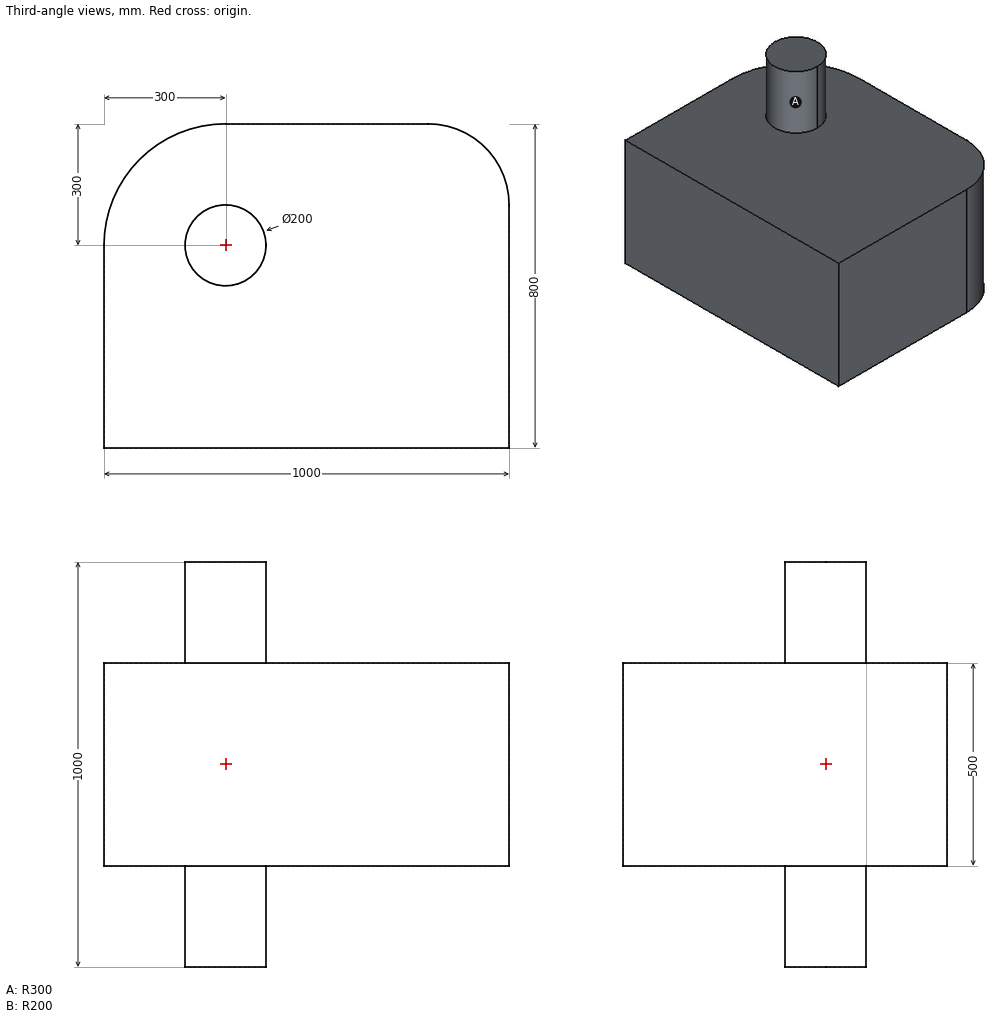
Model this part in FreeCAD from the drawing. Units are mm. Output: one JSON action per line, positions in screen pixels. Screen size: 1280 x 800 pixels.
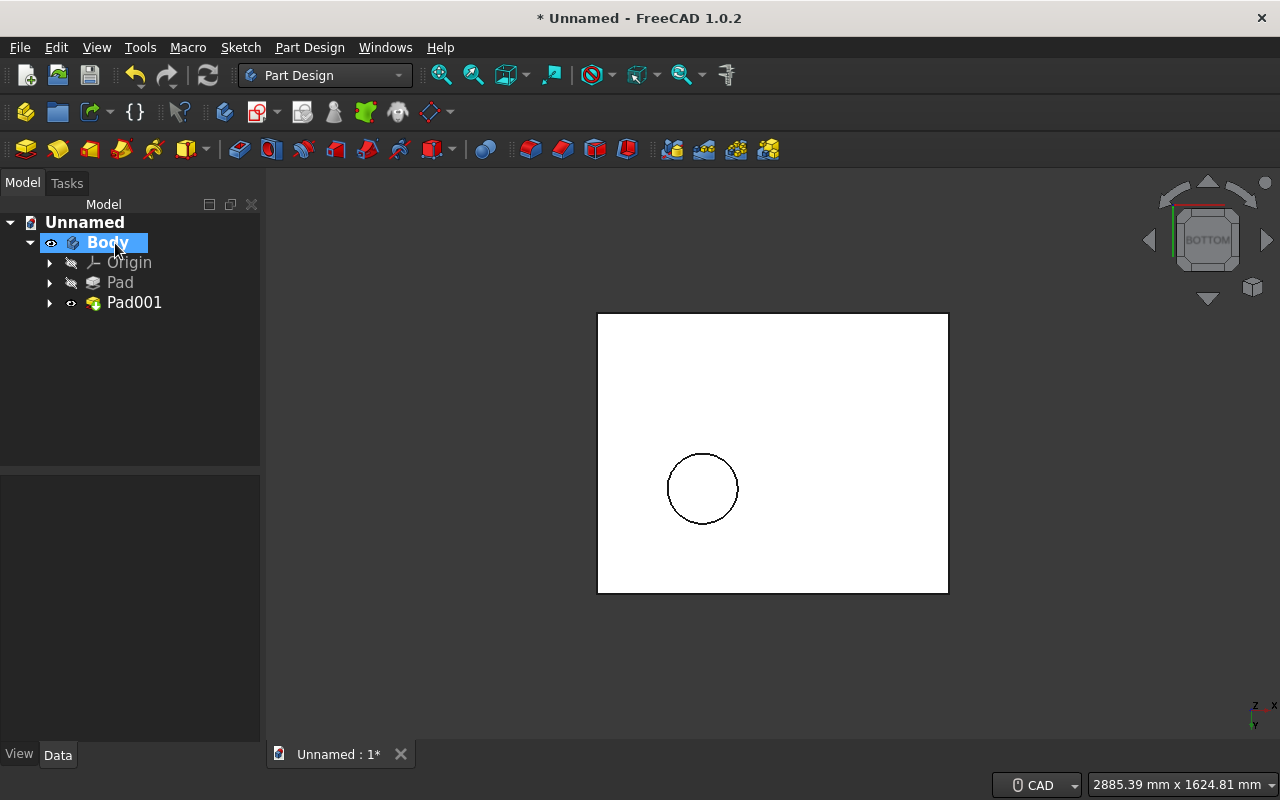
{"action": "key", "text": "4"}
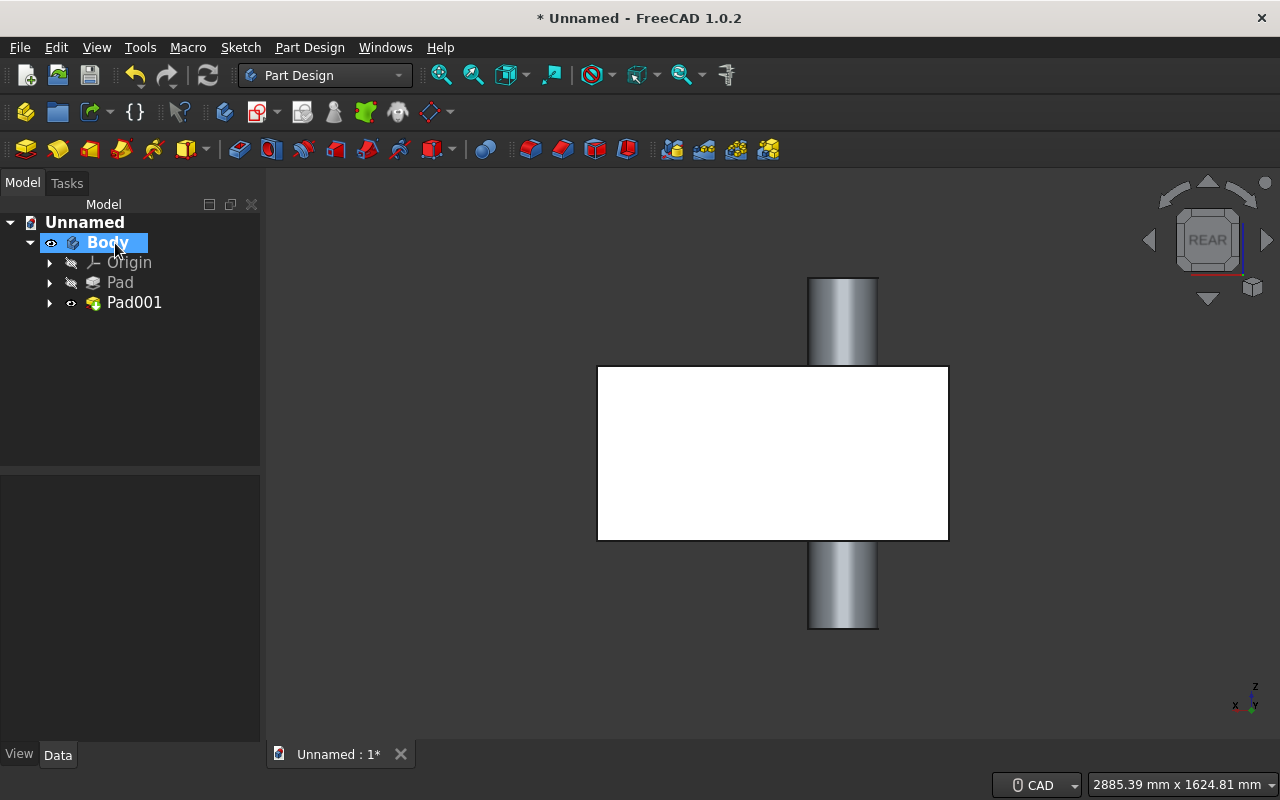
{"action": "left_click", "coordinate": [949, 452]}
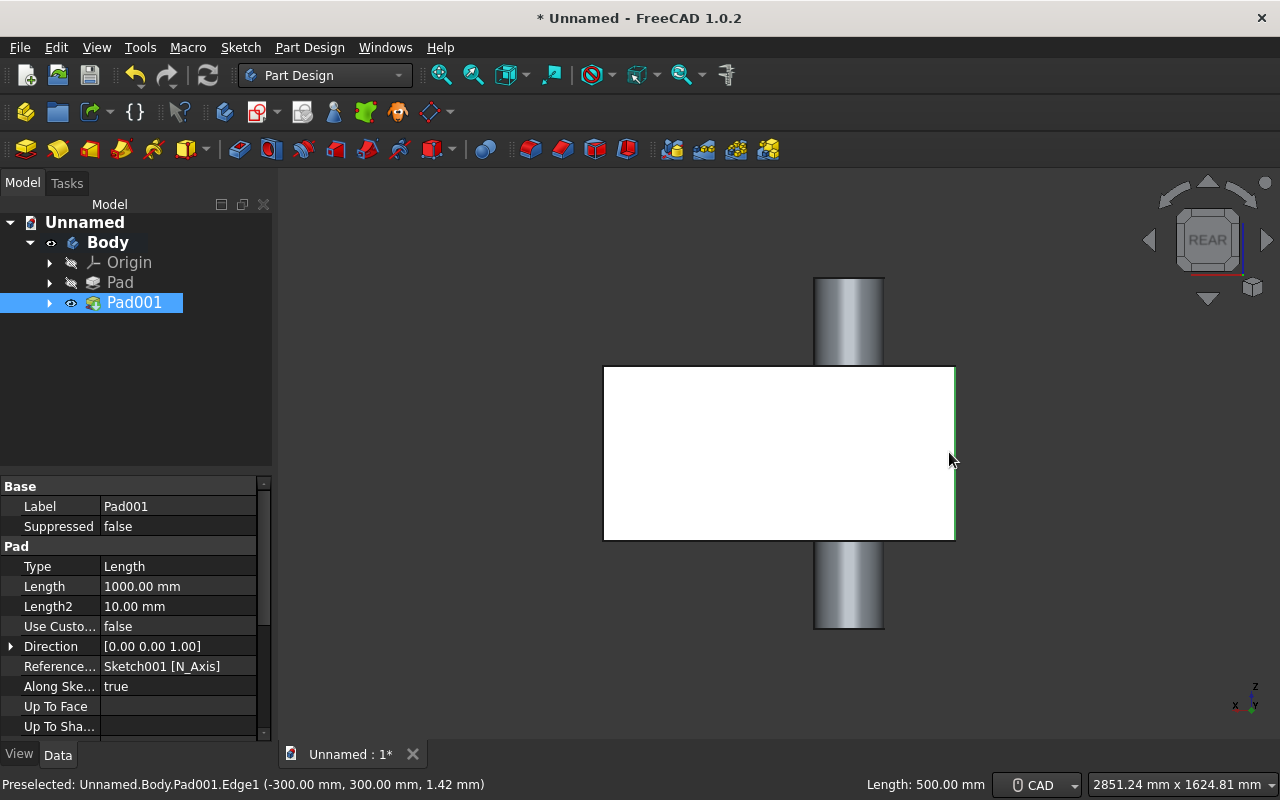
{"action": "left_click", "coordinate": [532, 150]}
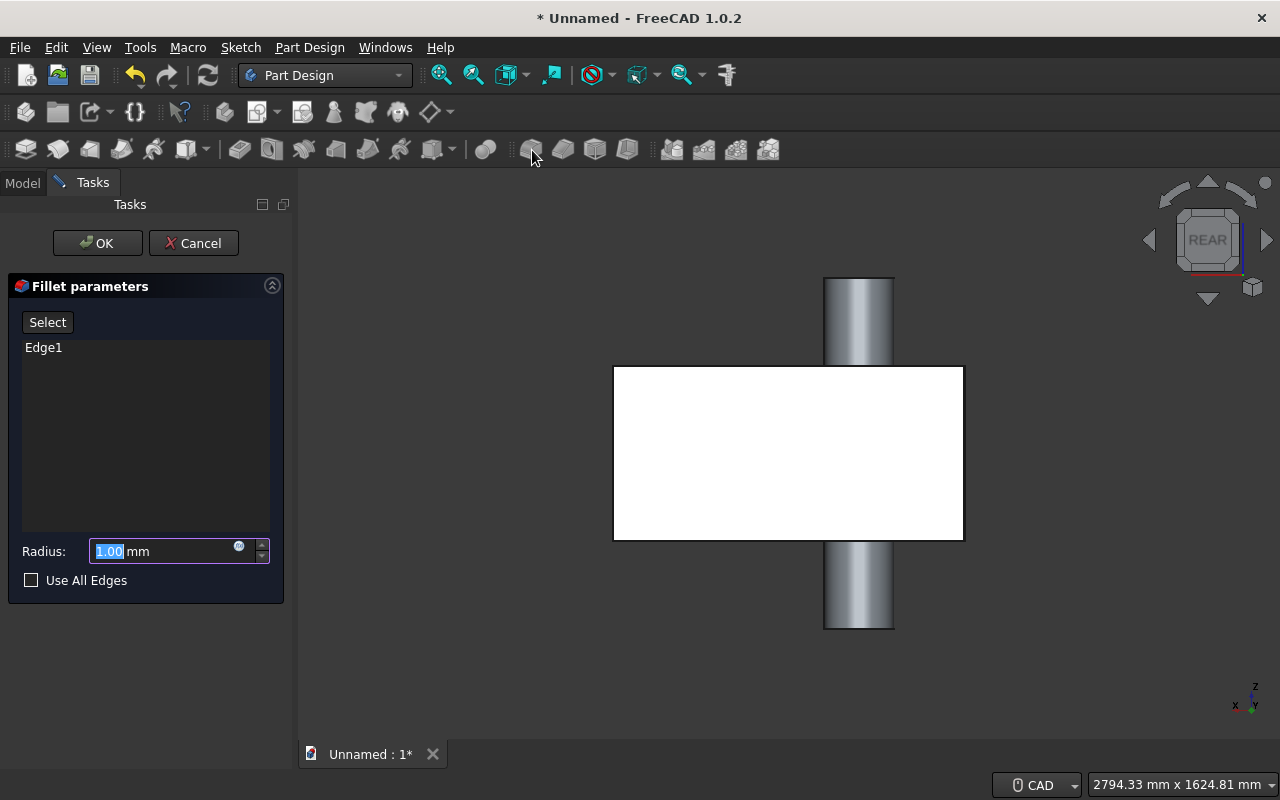
{"action": "type", "text": "300"}
{"action": "key", "text": "Tab"}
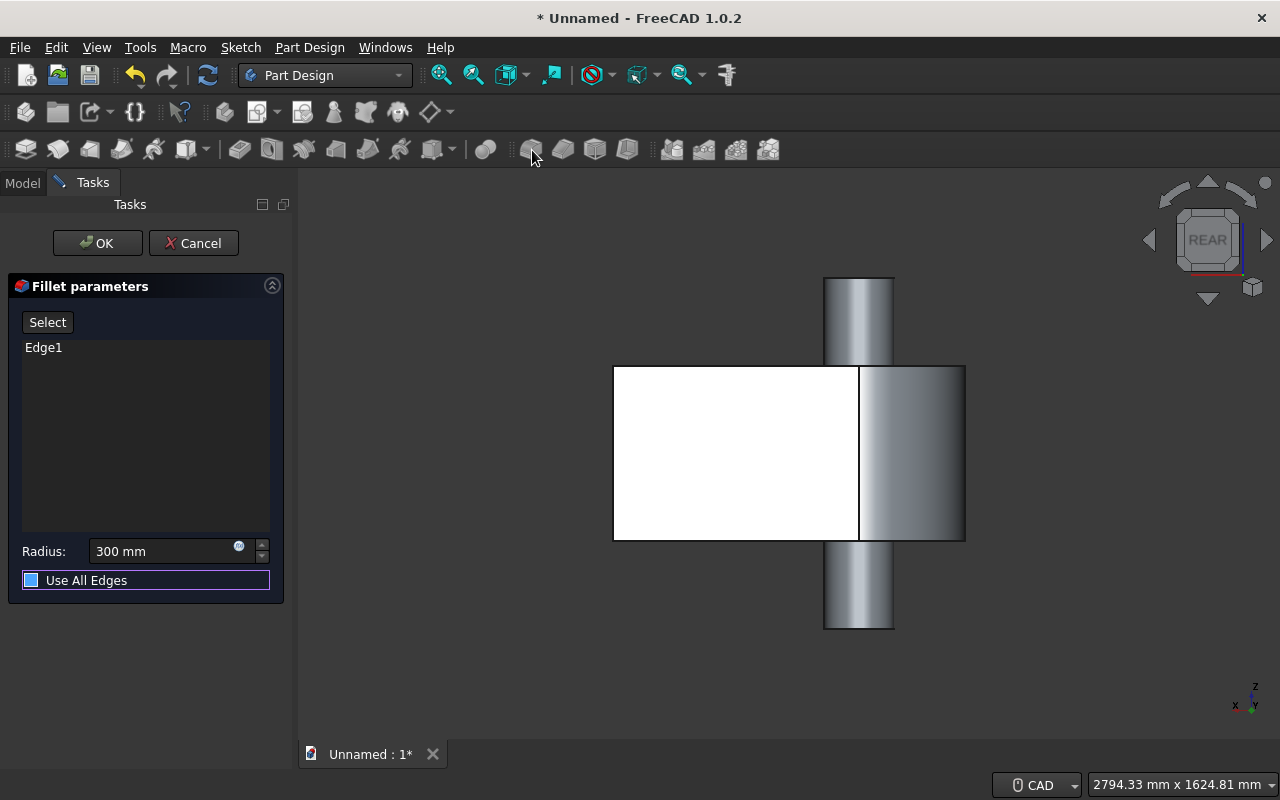
{"action": "left_click", "coordinate": [98, 243]}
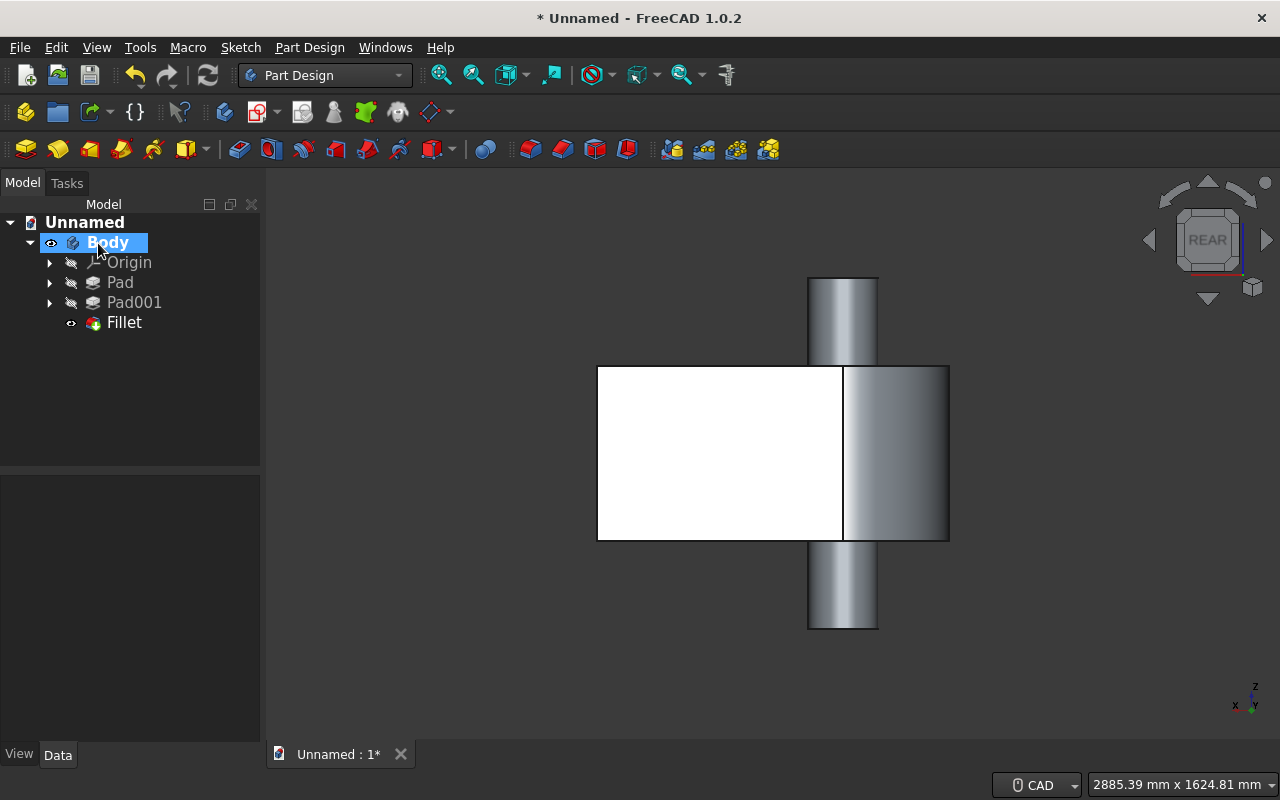
{"action": "left_click", "coordinate": [597, 452]}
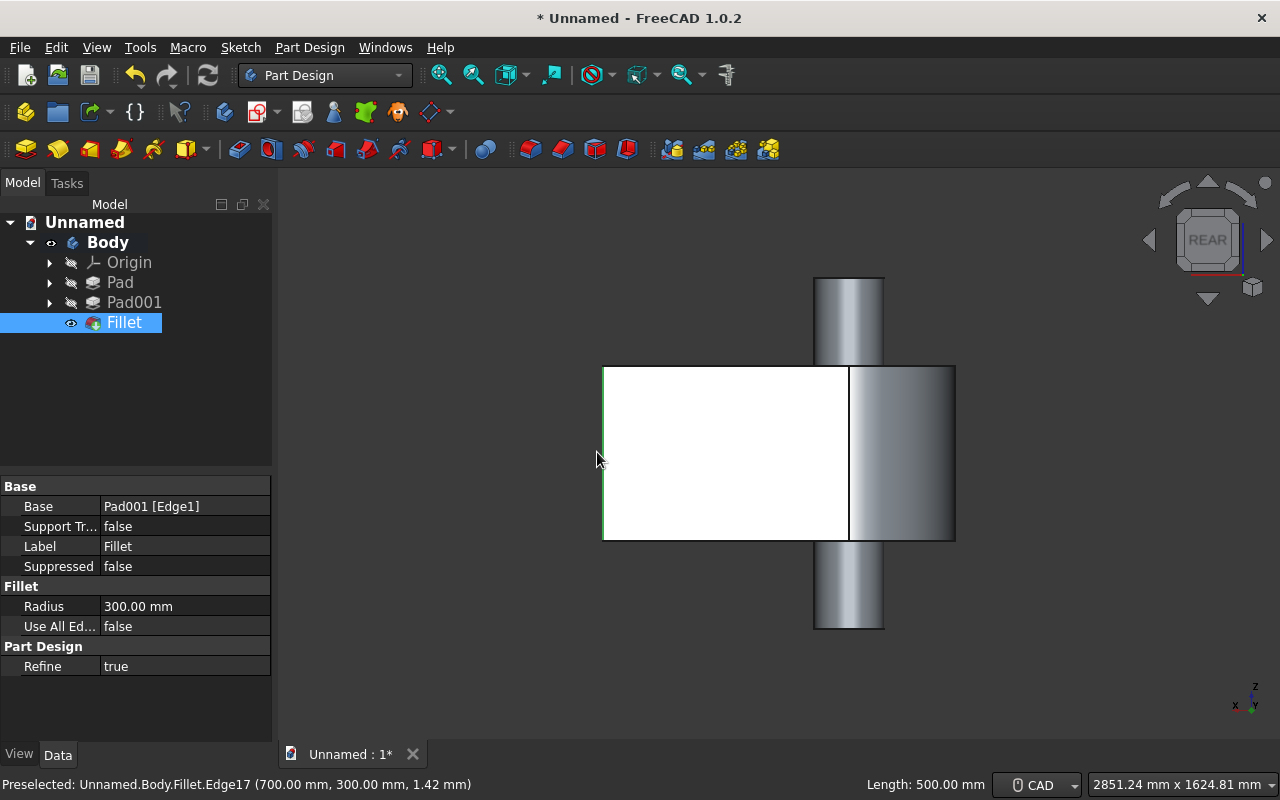
{"action": "left_click", "coordinate": [532, 150]}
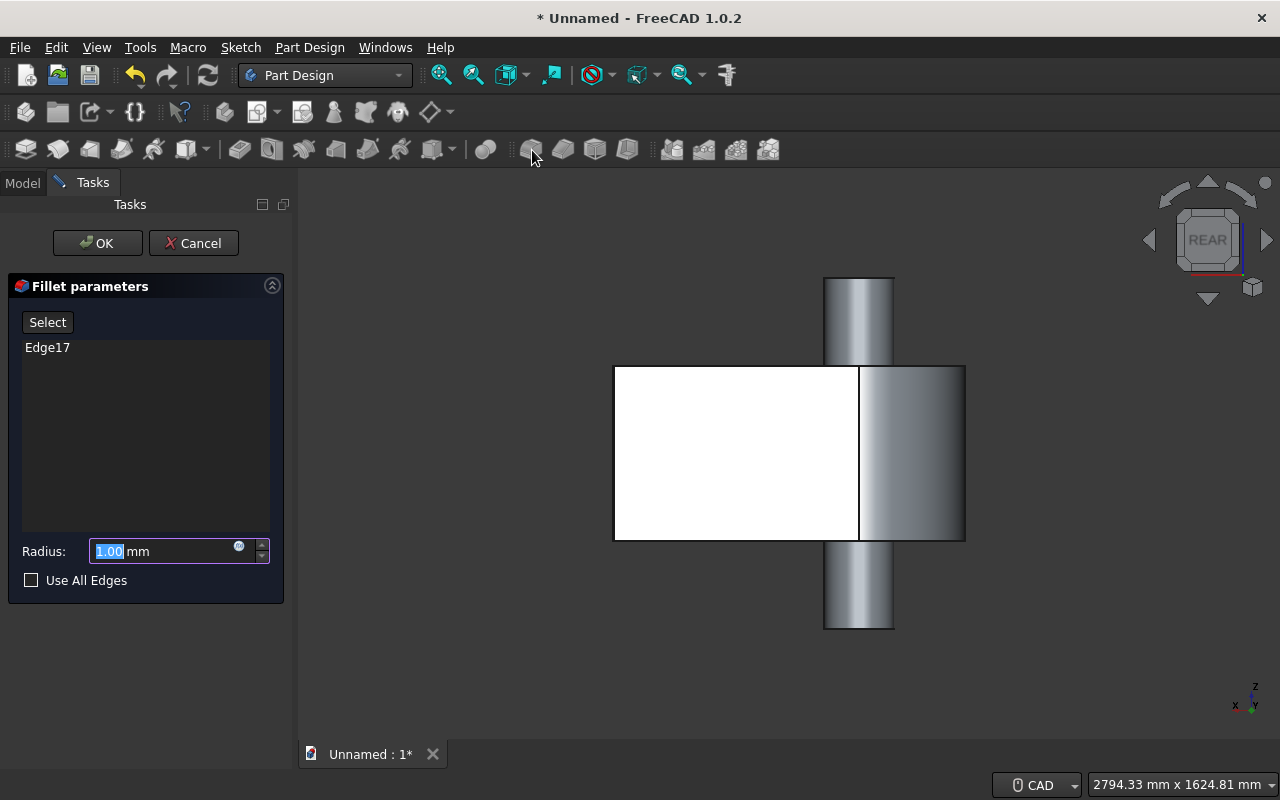
{"action": "type", "text": "200"}
{"action": "key", "text": "Tab"}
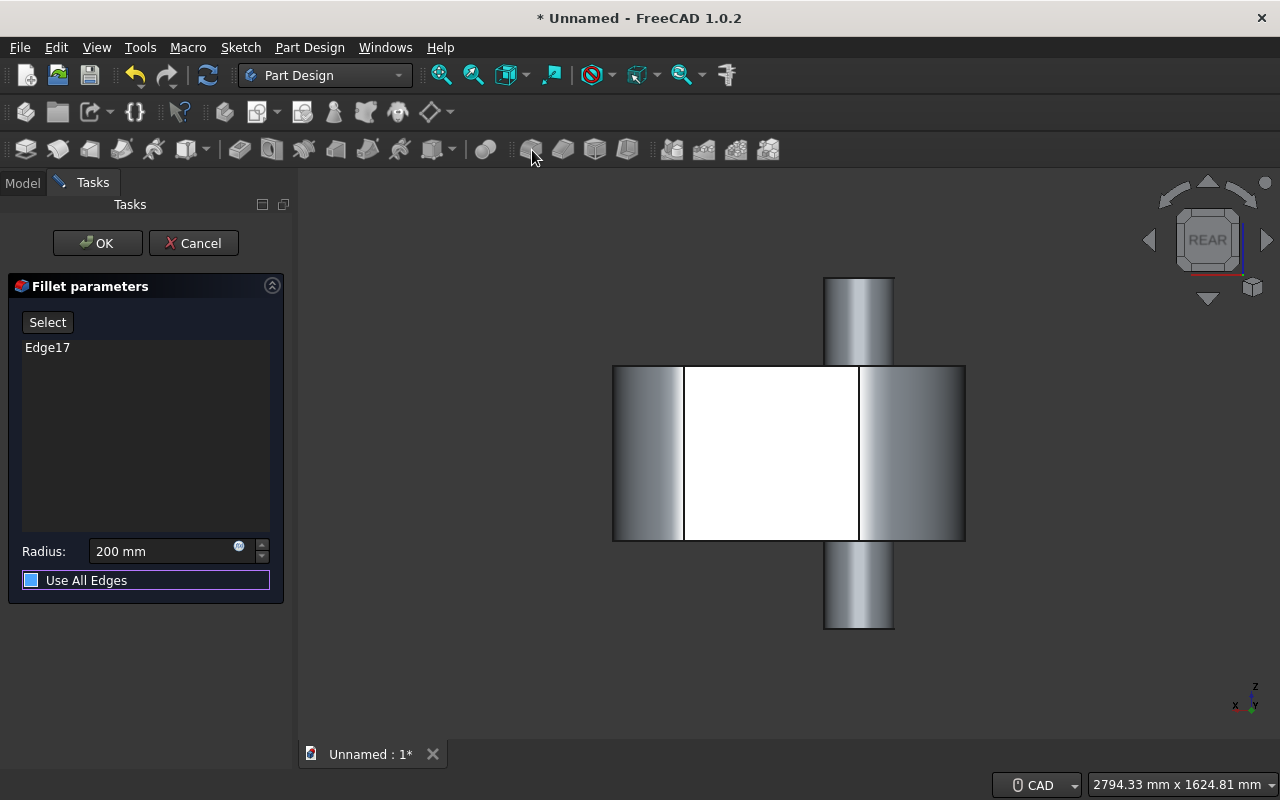
{"action": "left_click", "coordinate": [98, 243]}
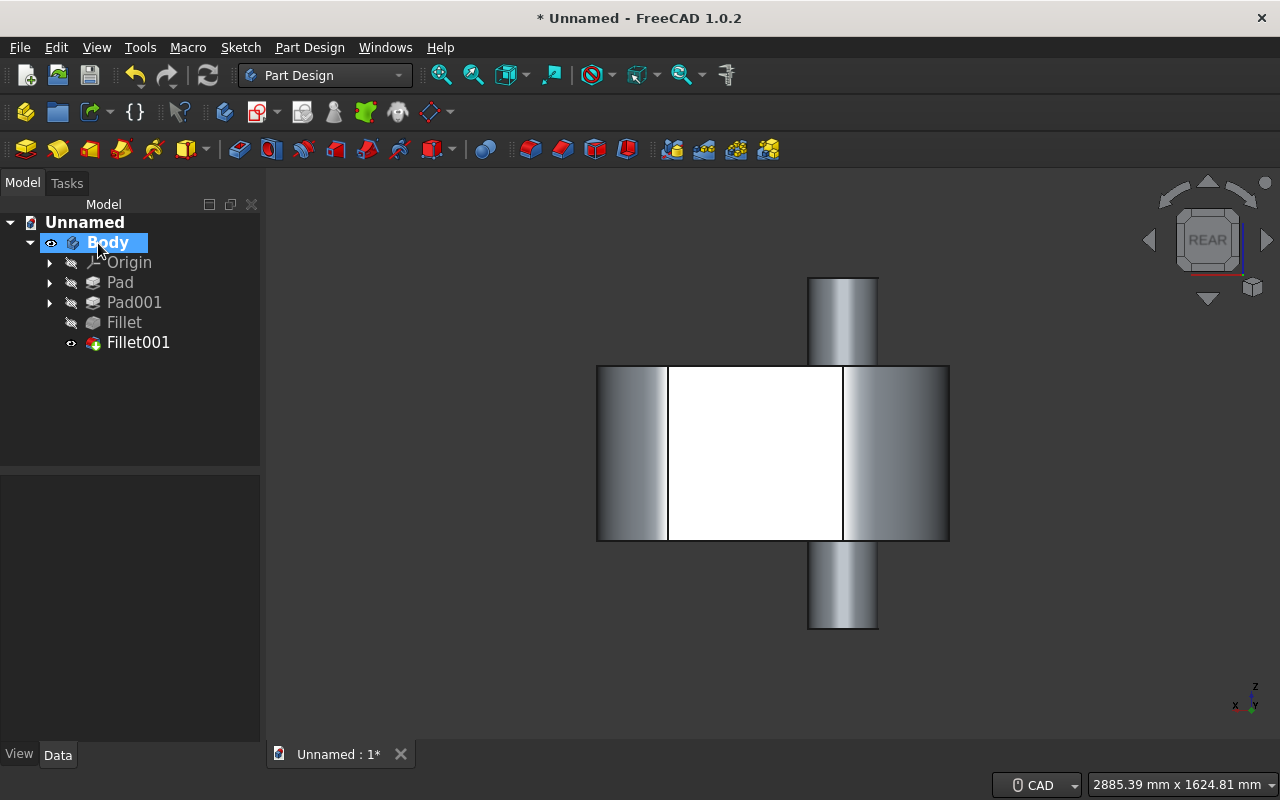
{"action": "key", "text": "0"}